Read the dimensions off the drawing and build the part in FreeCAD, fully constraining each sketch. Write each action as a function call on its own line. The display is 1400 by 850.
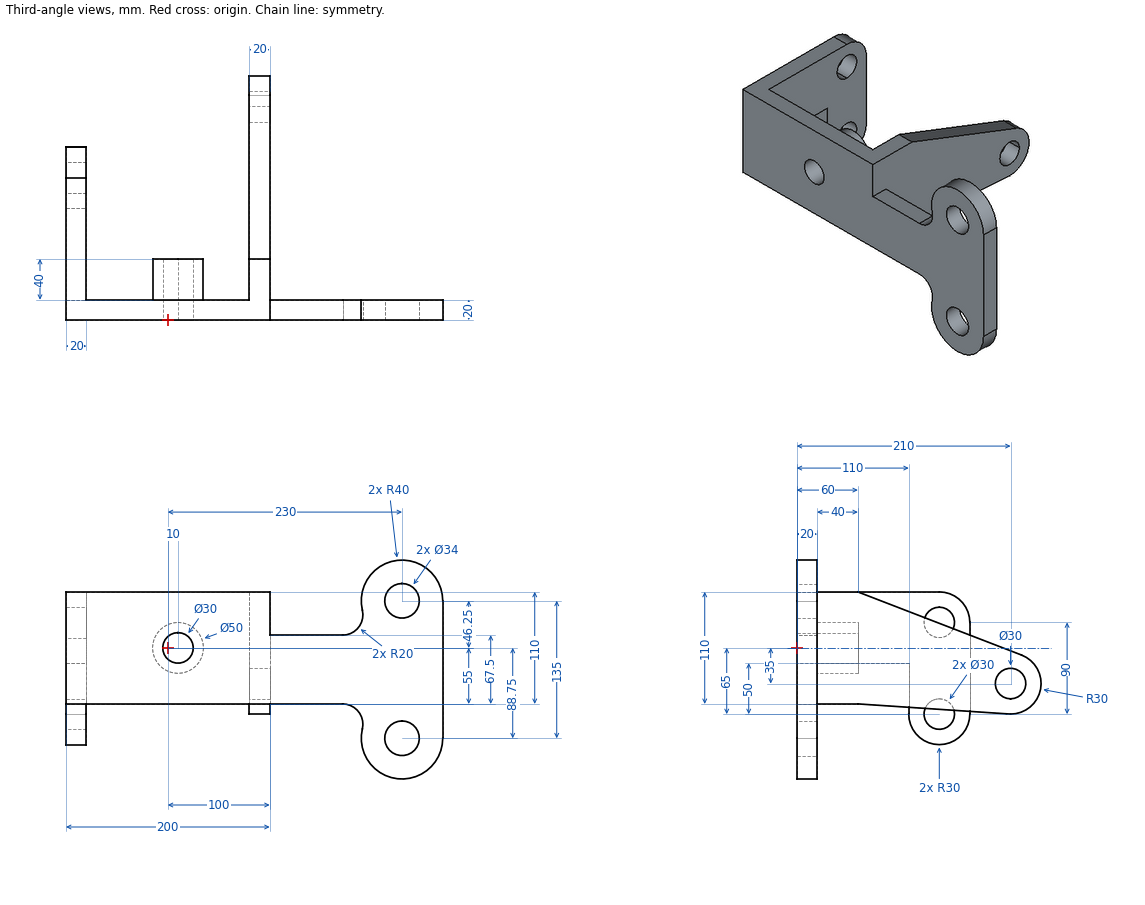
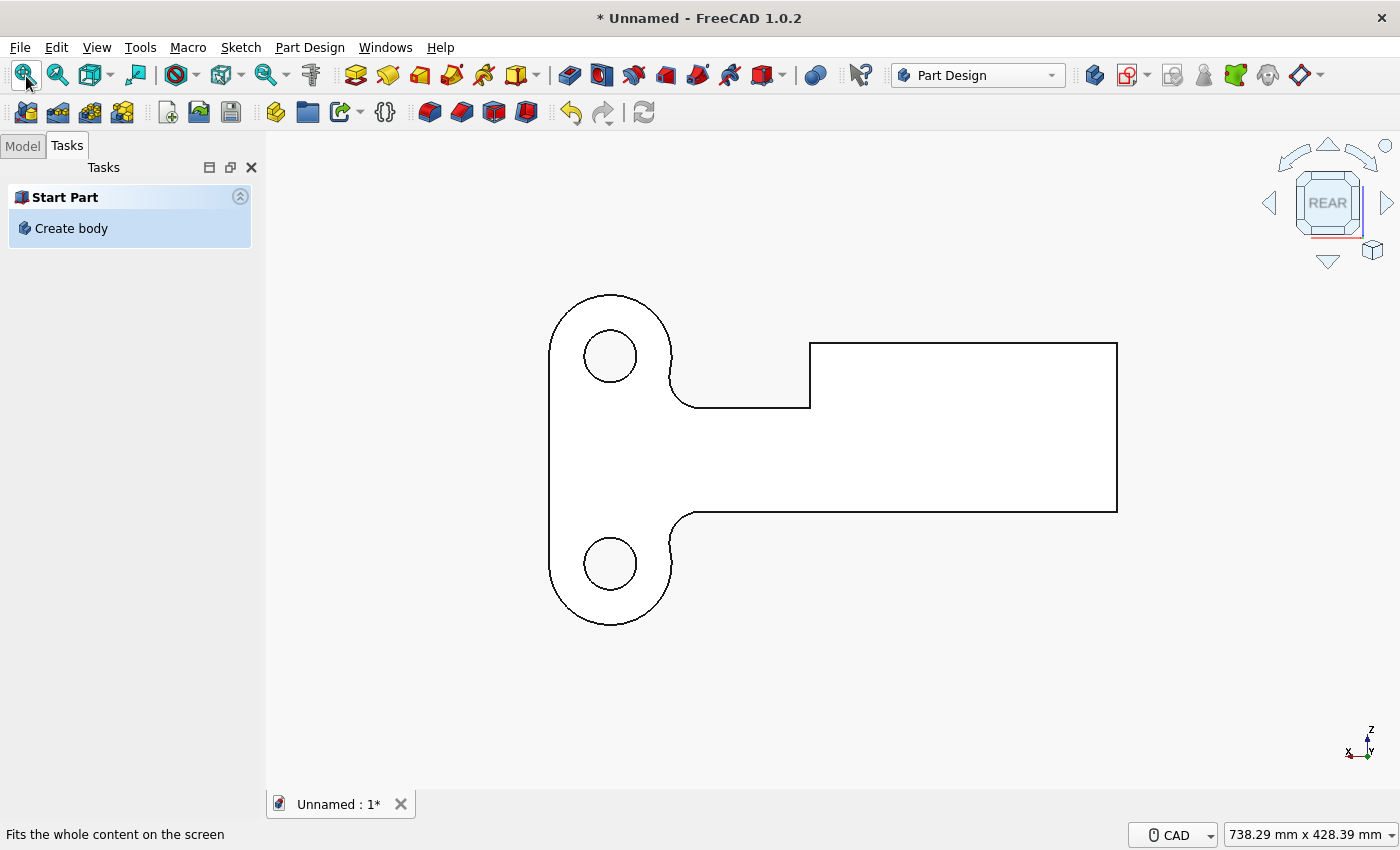
key(6)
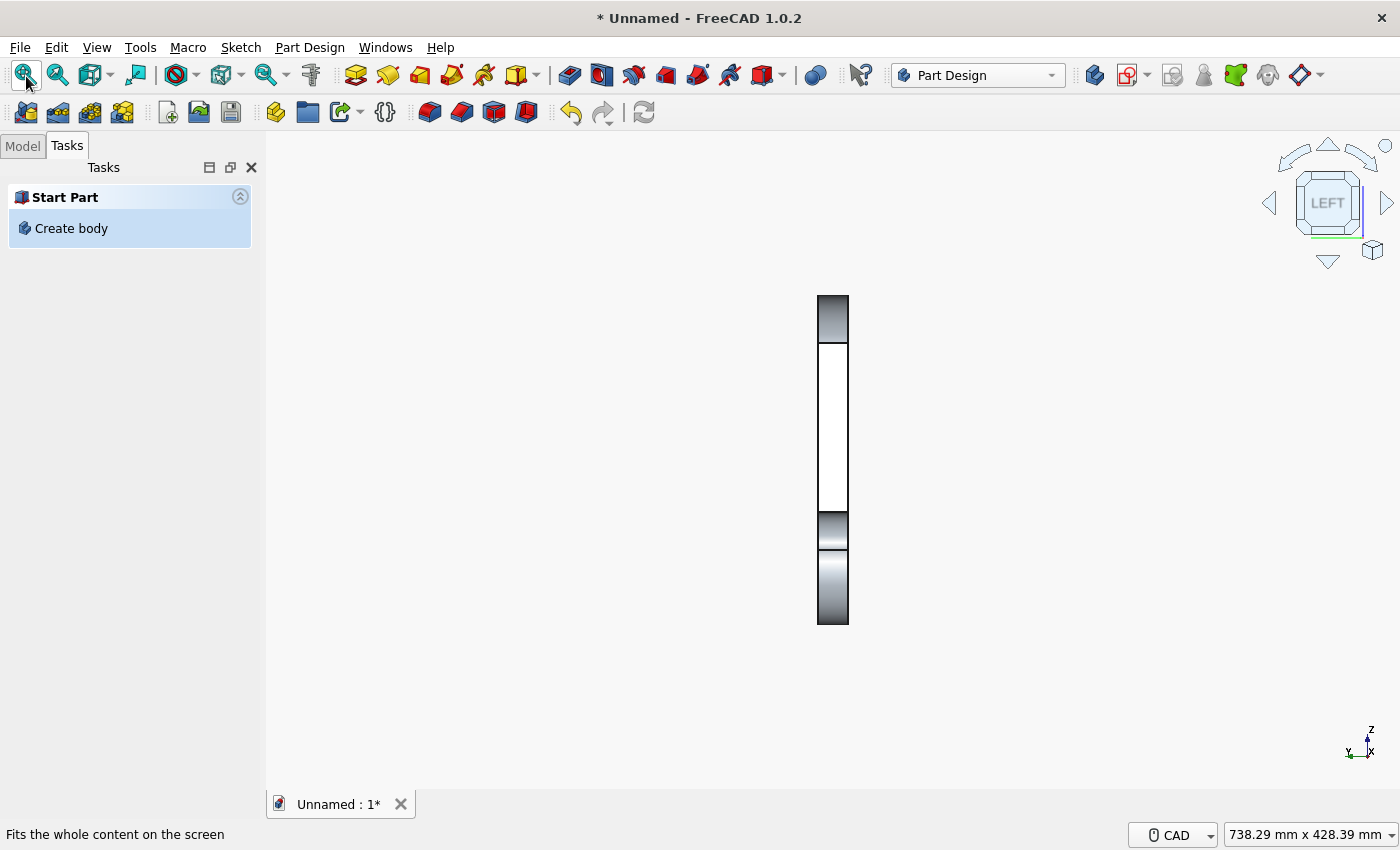
click(833, 426)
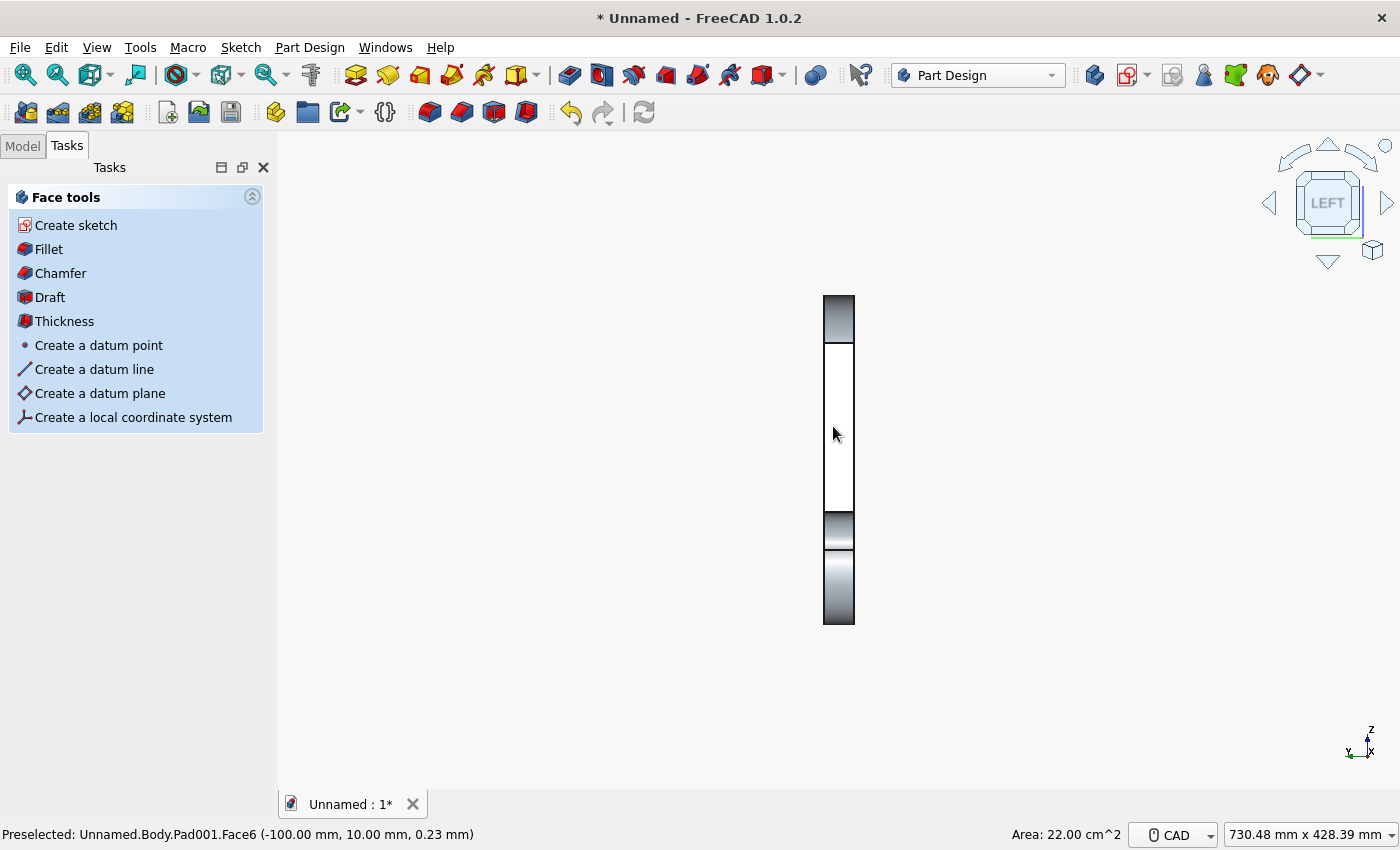
click(1128, 76)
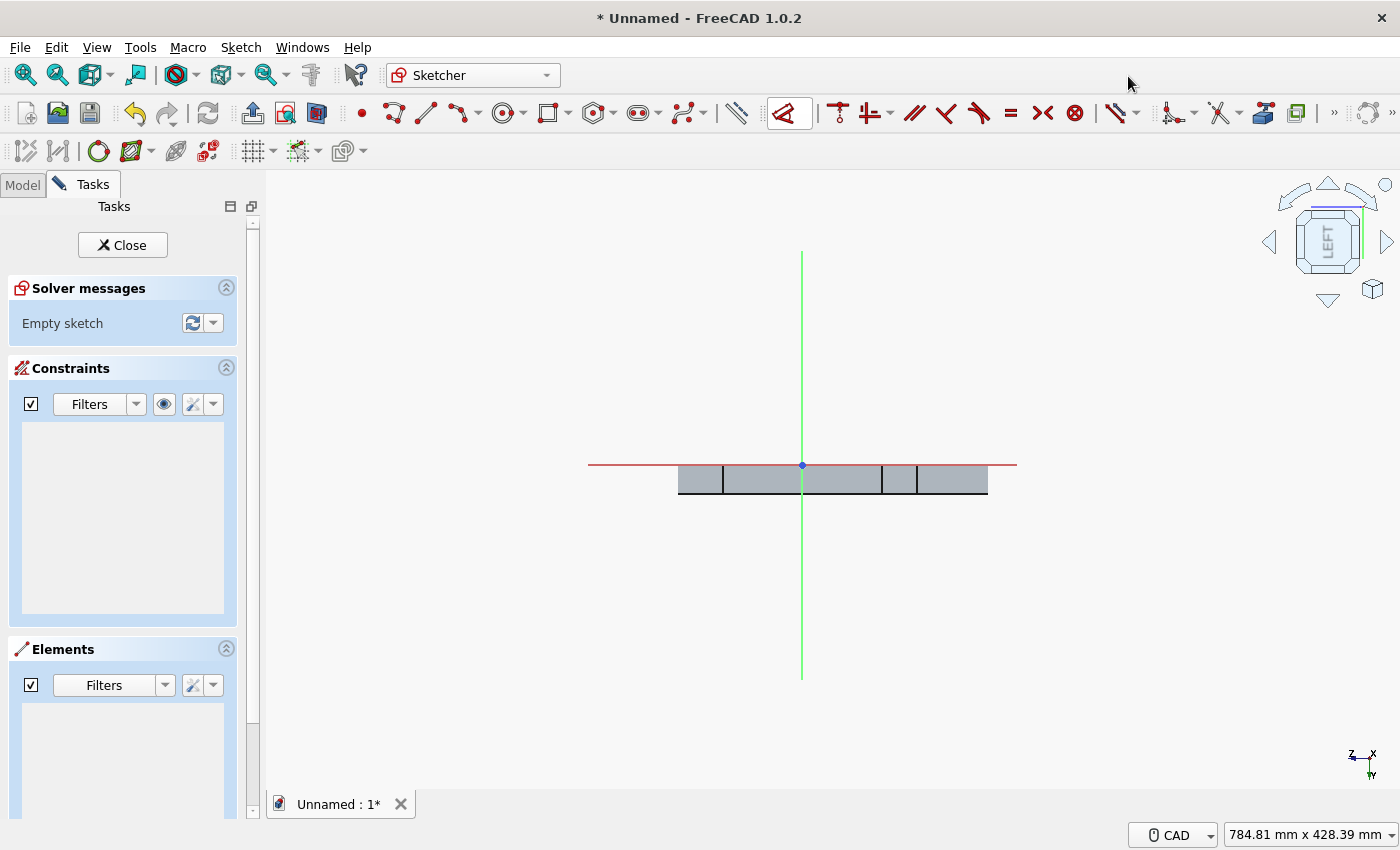
scroll(967, 761, up, 2)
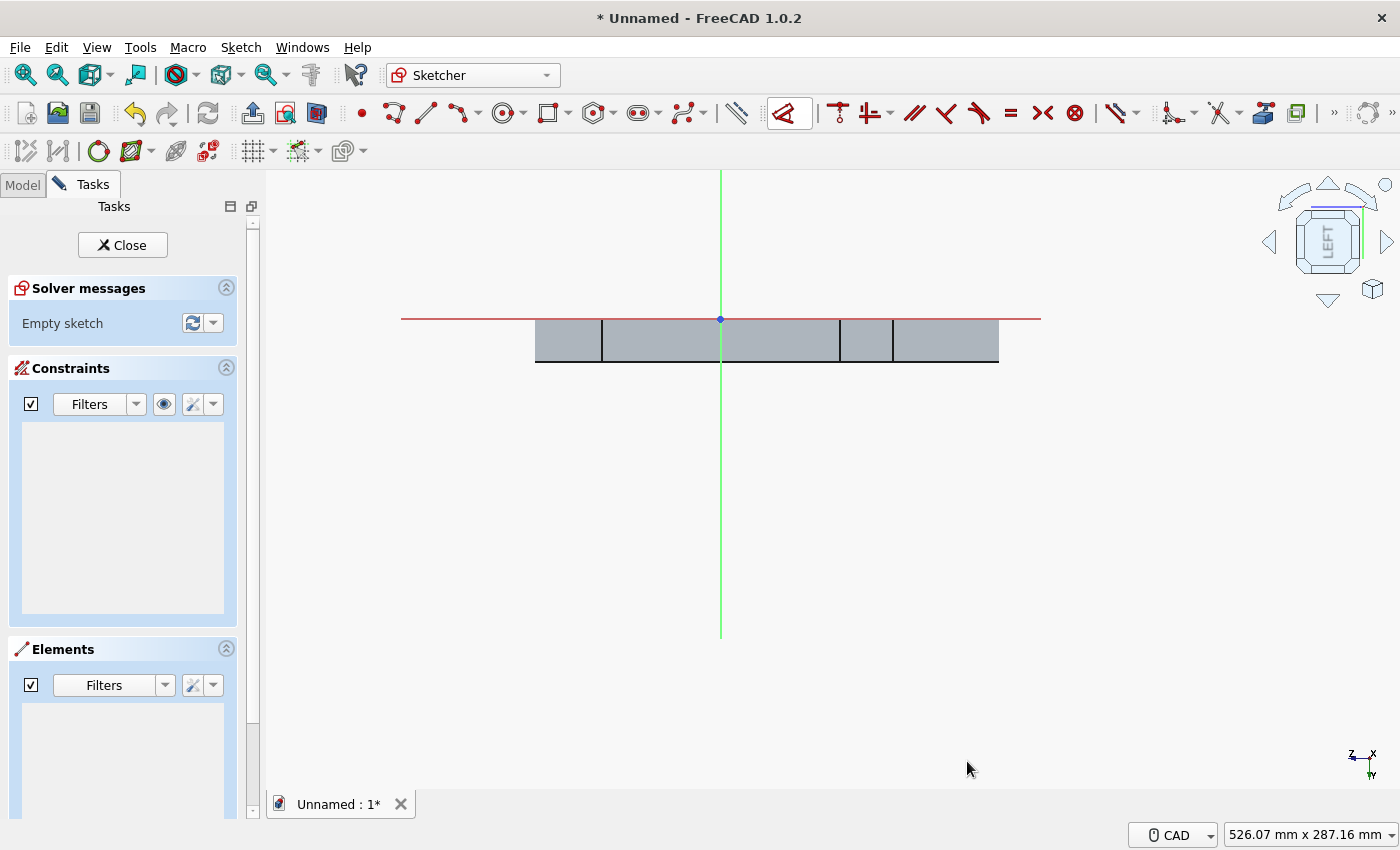
key(g)
key(l)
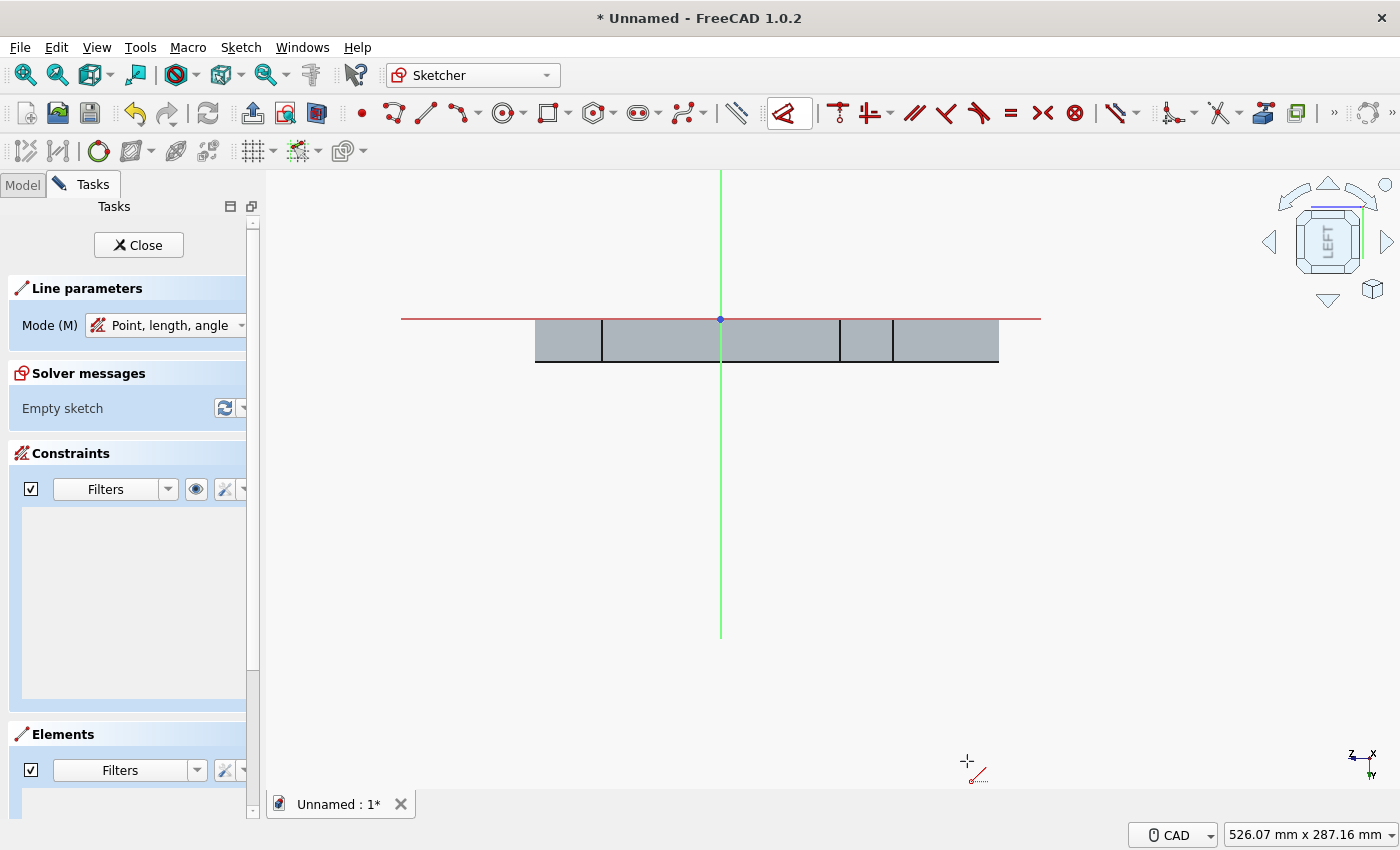
click(667, 685)
click(861, 685)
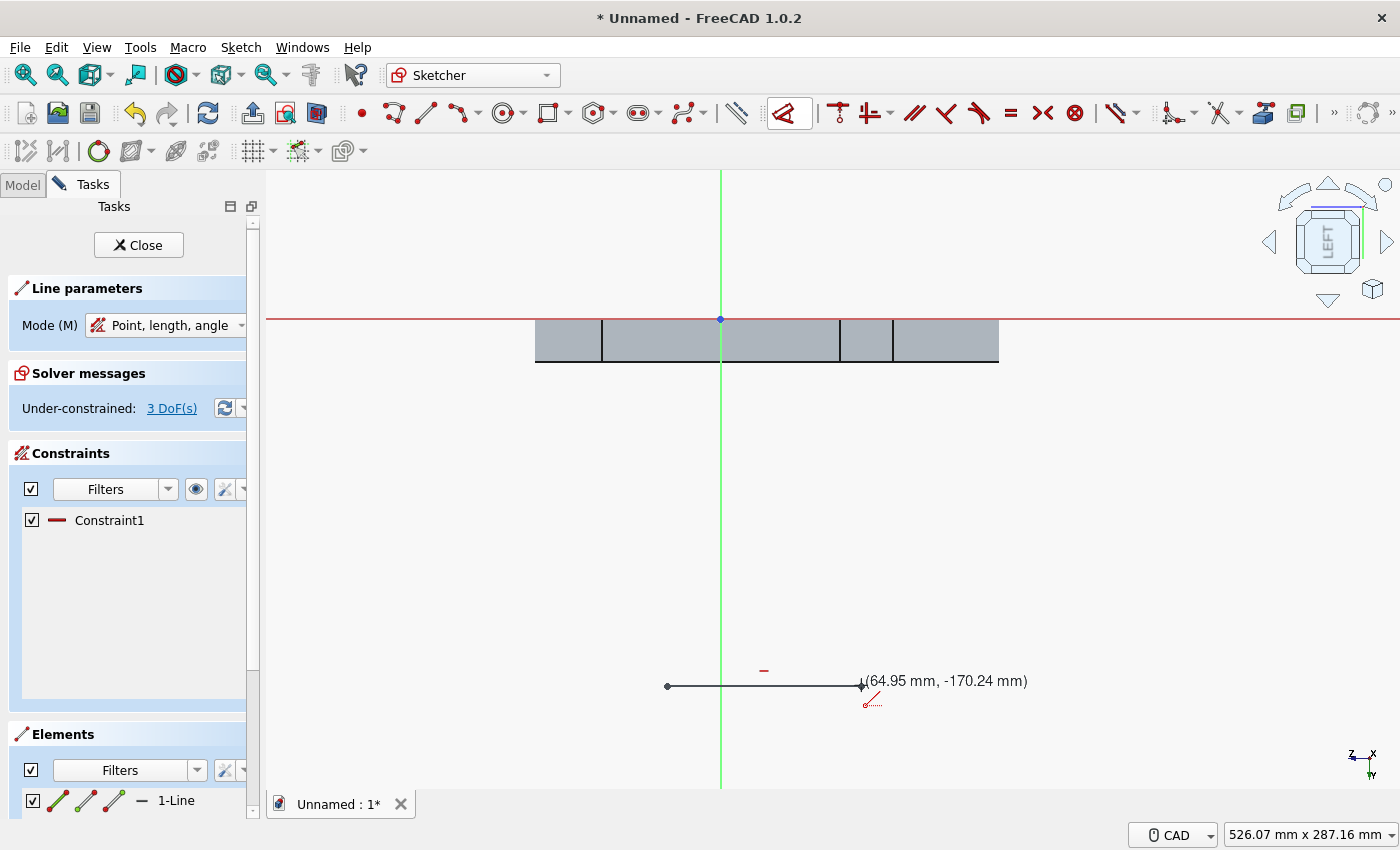
key(g)
key(m)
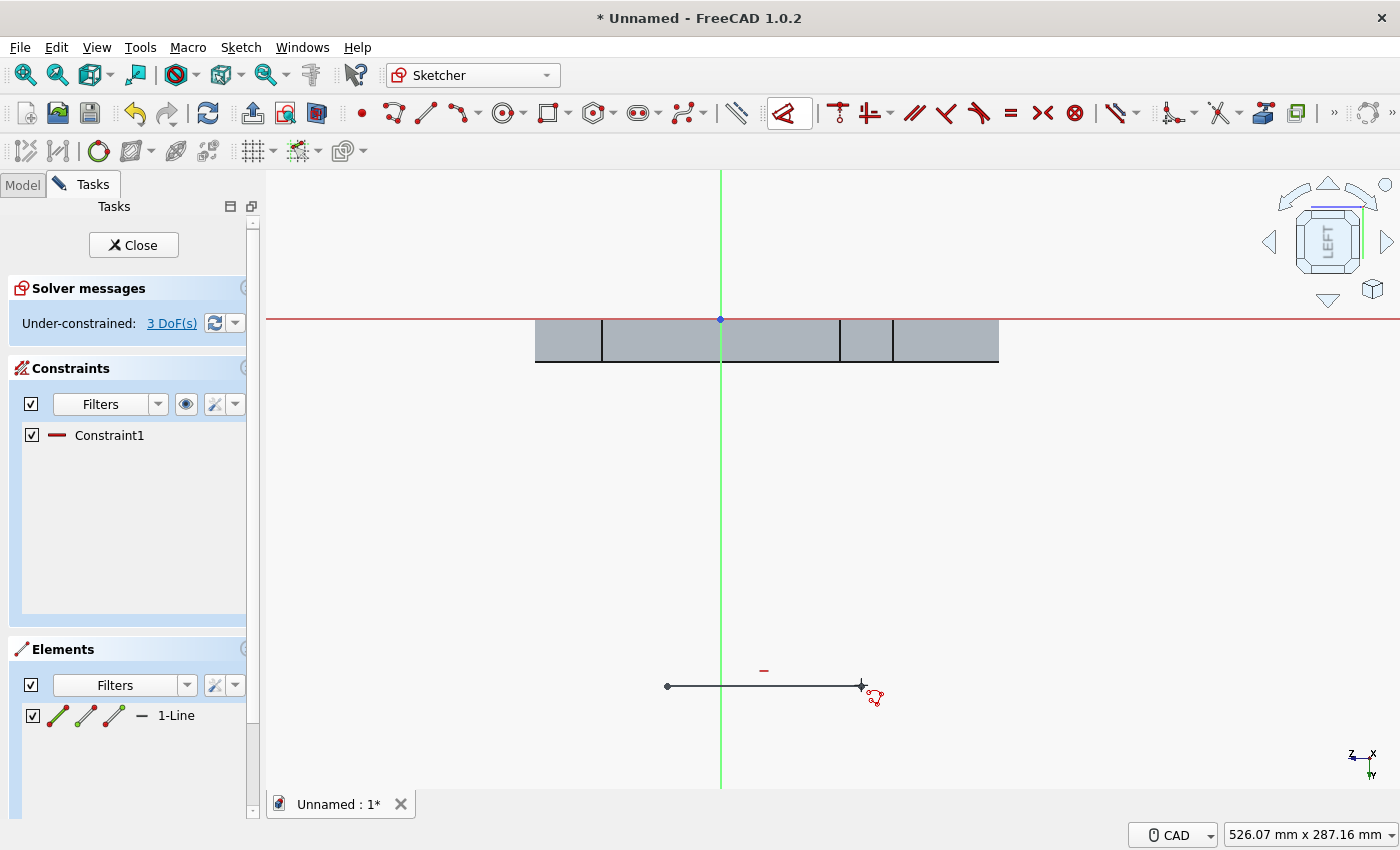
click(861, 556)
click(753, 556)
click(753, 319)
click(602, 328)
click(602, 621)
right_click(602, 621)